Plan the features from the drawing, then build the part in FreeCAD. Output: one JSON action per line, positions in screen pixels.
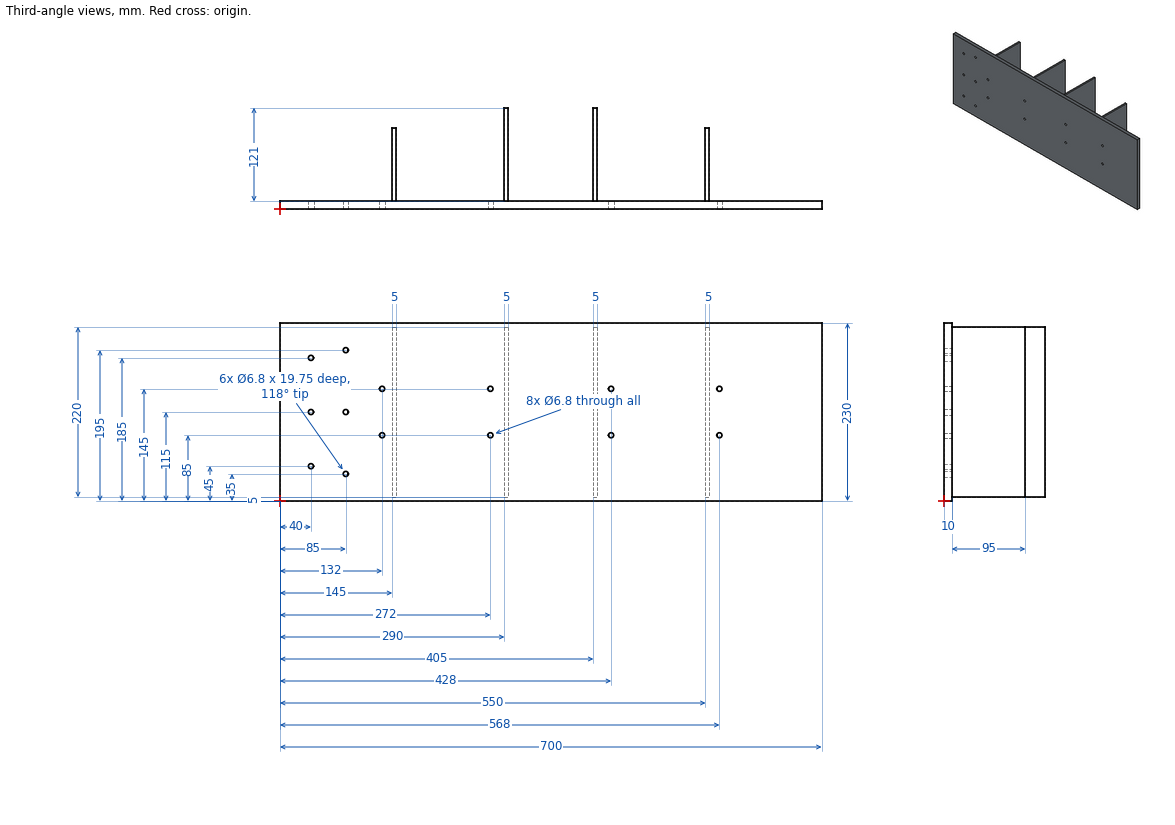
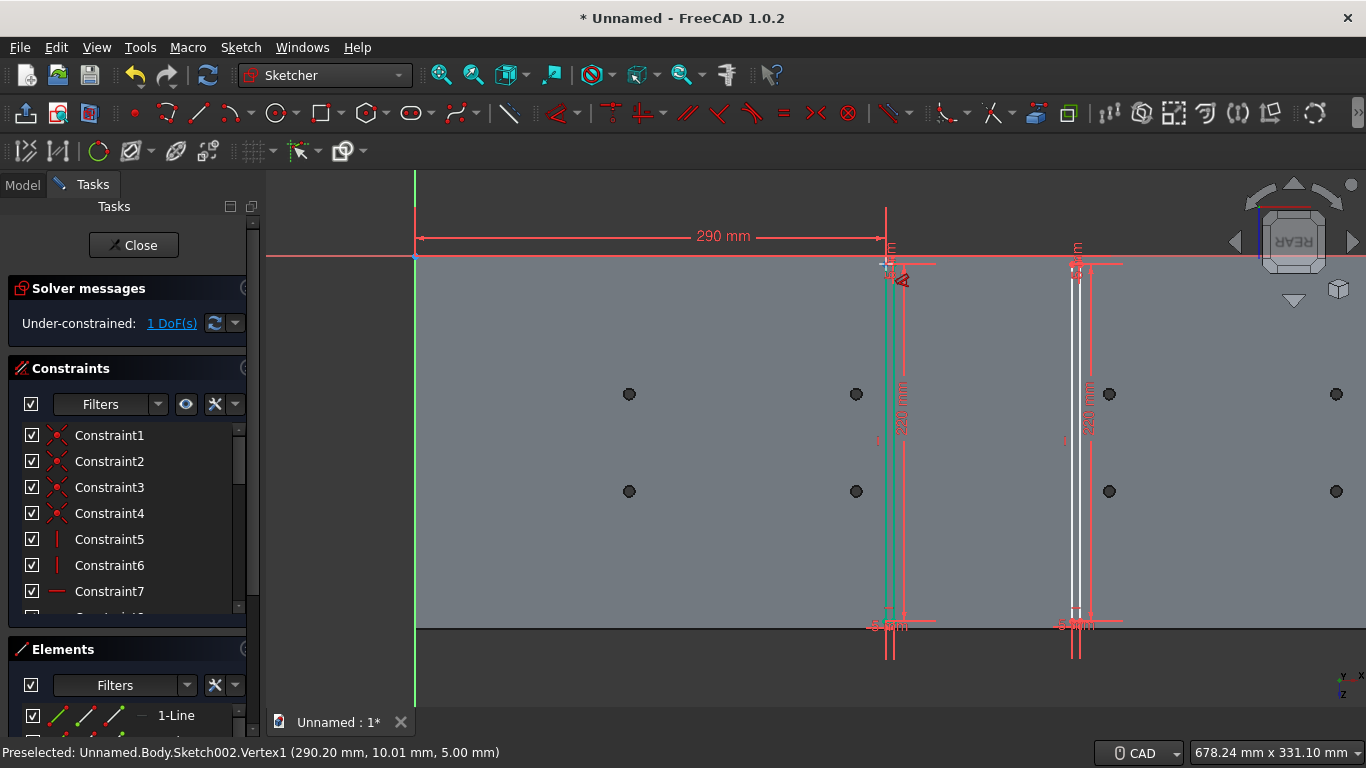
{"action": "scroll", "coordinate": [1072, 264], "scroll_direction": "up", "scroll_amount": 3}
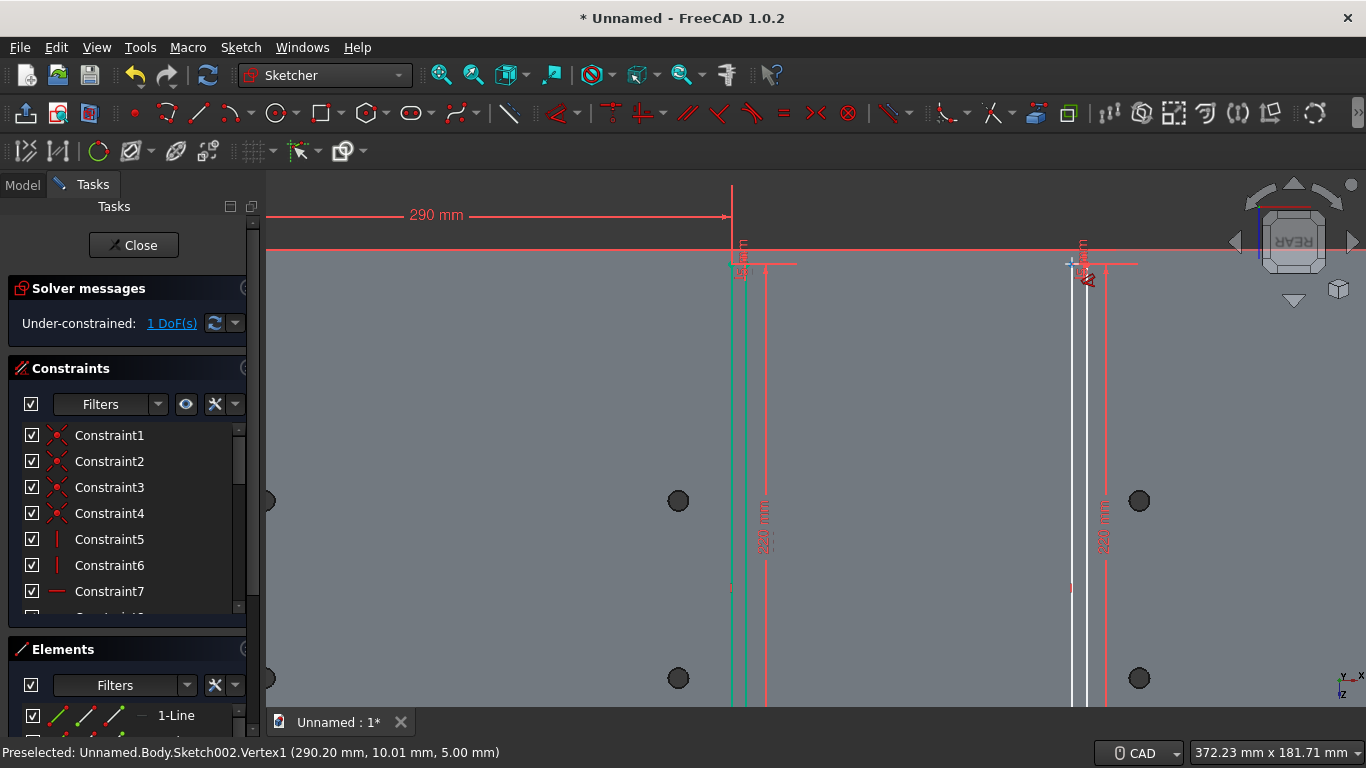
{"action": "left_click", "coordinate": [1072, 264]}
{"action": "left_click", "coordinate": [683, 216]}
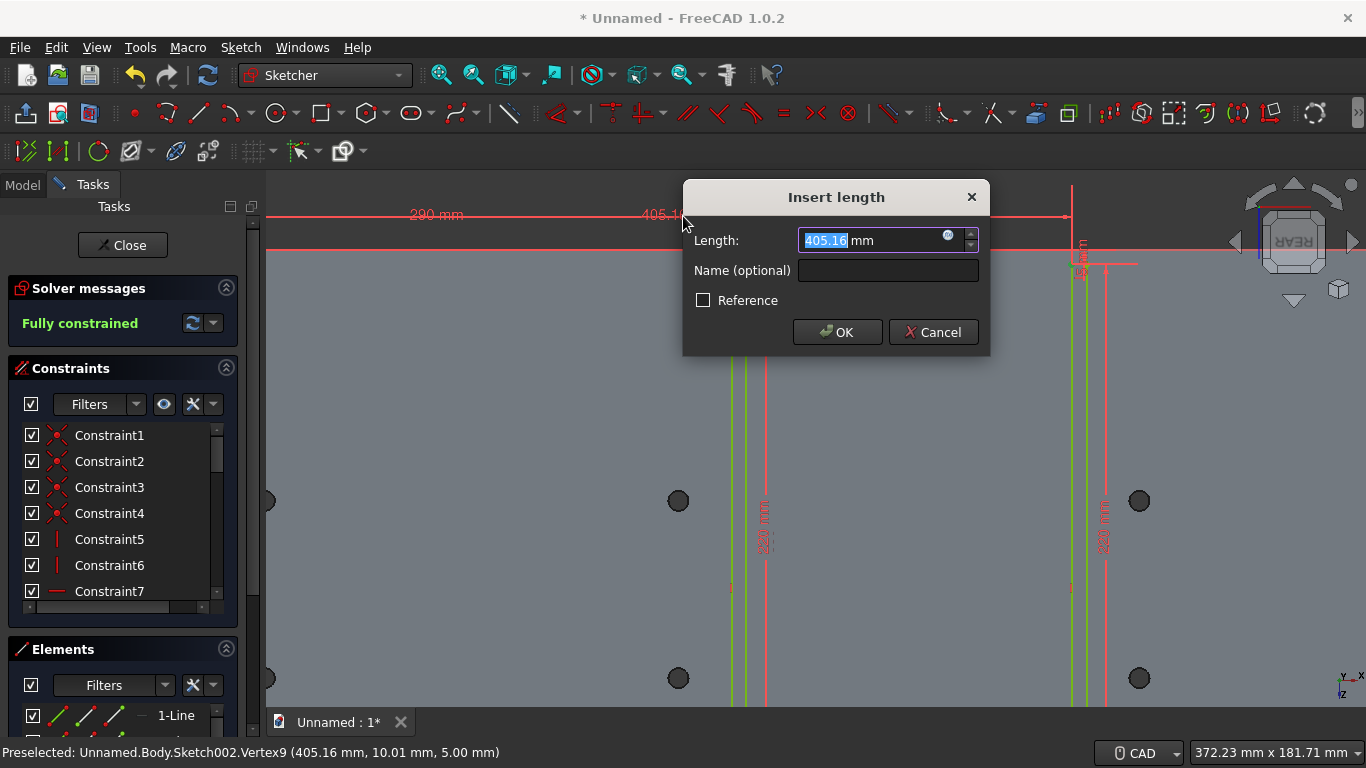
{"action": "type", "text": "405"}
{"action": "key", "text": "Return"}
{"action": "key", "text": "Escape"}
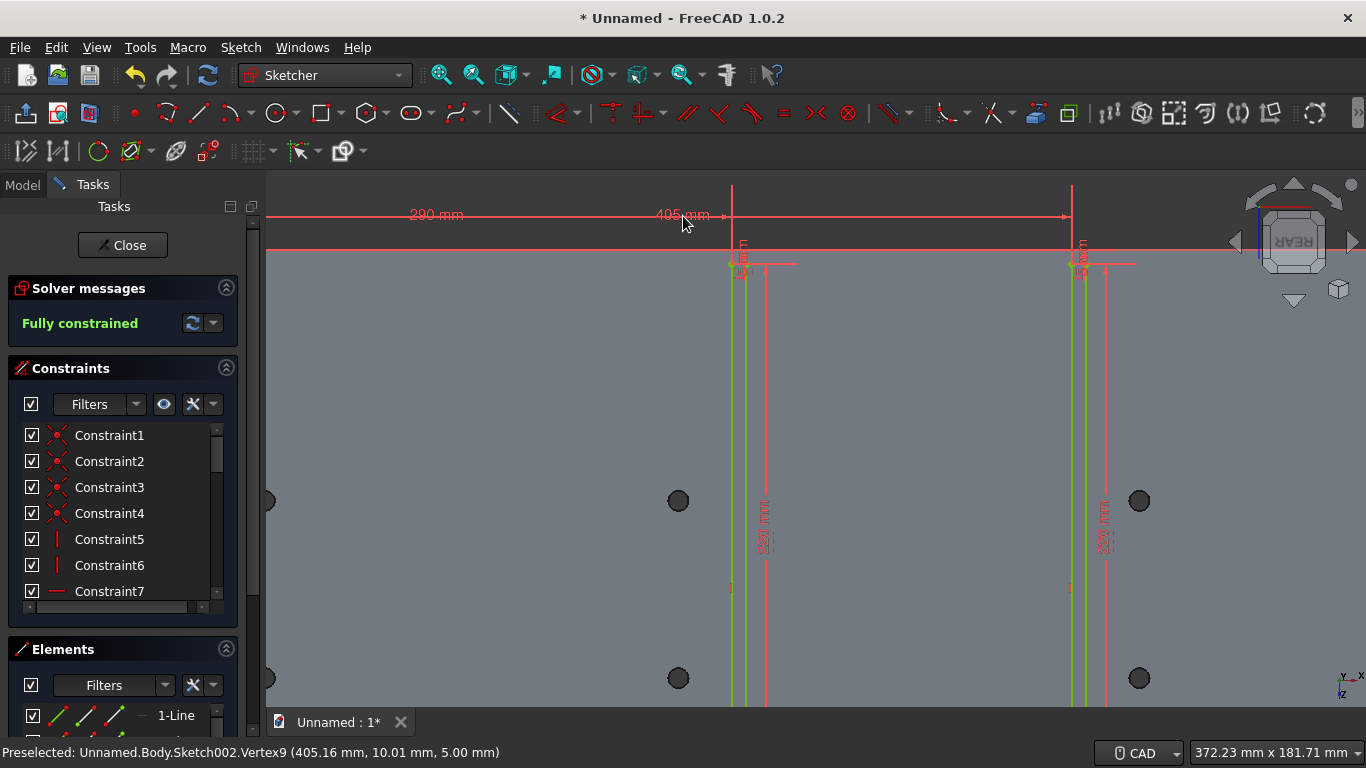
{"action": "left_click", "coordinate": [123, 245]}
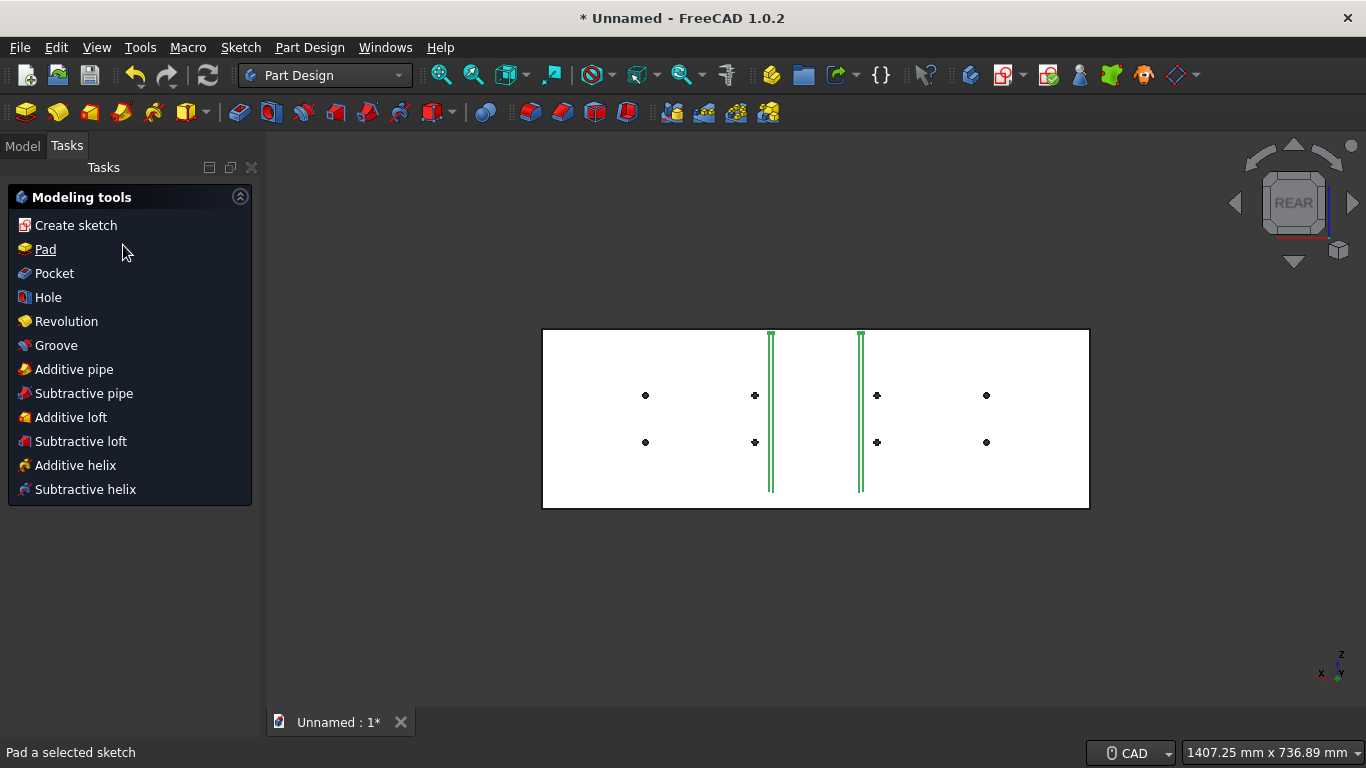
{"action": "left_click", "coordinate": [26, 112]}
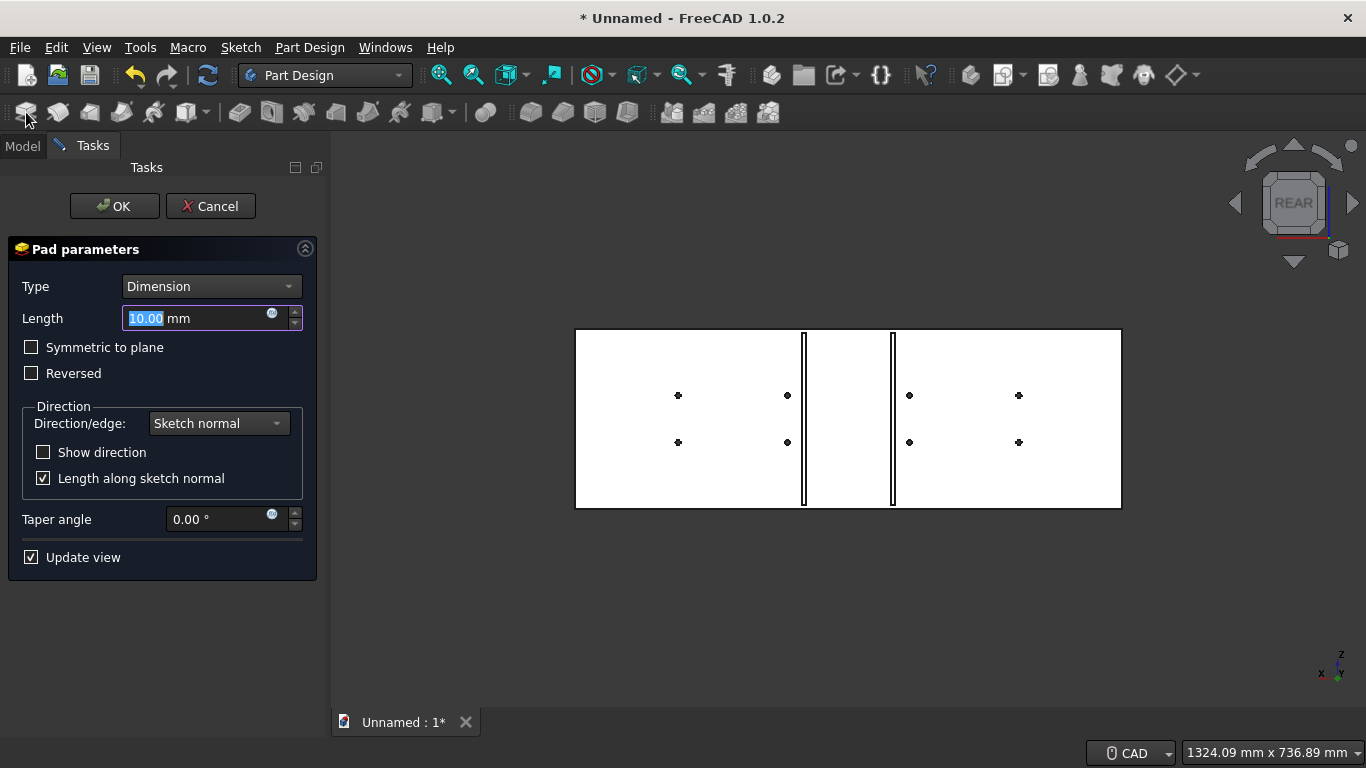
{"action": "type", "text": "121"}
{"action": "key", "text": "Tab"}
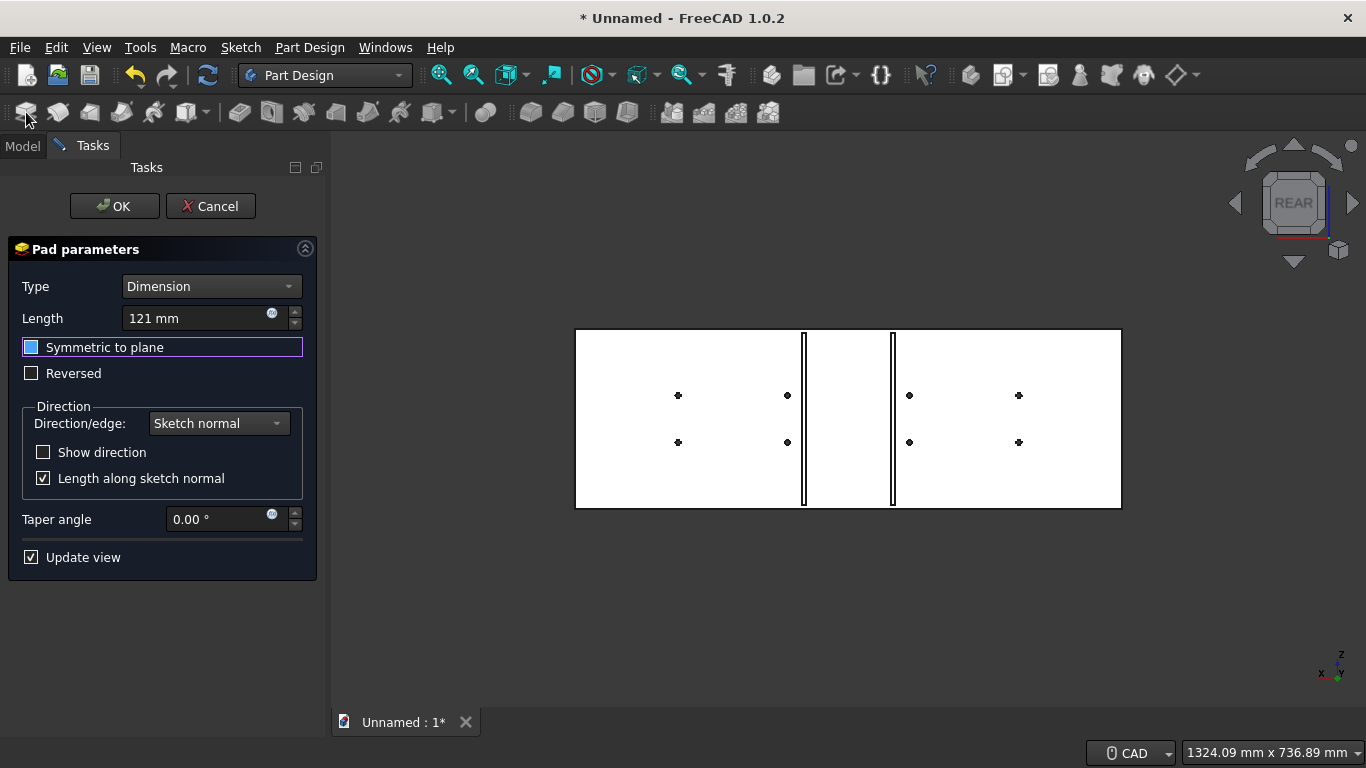
{"action": "left_click", "coordinate": [115, 206]}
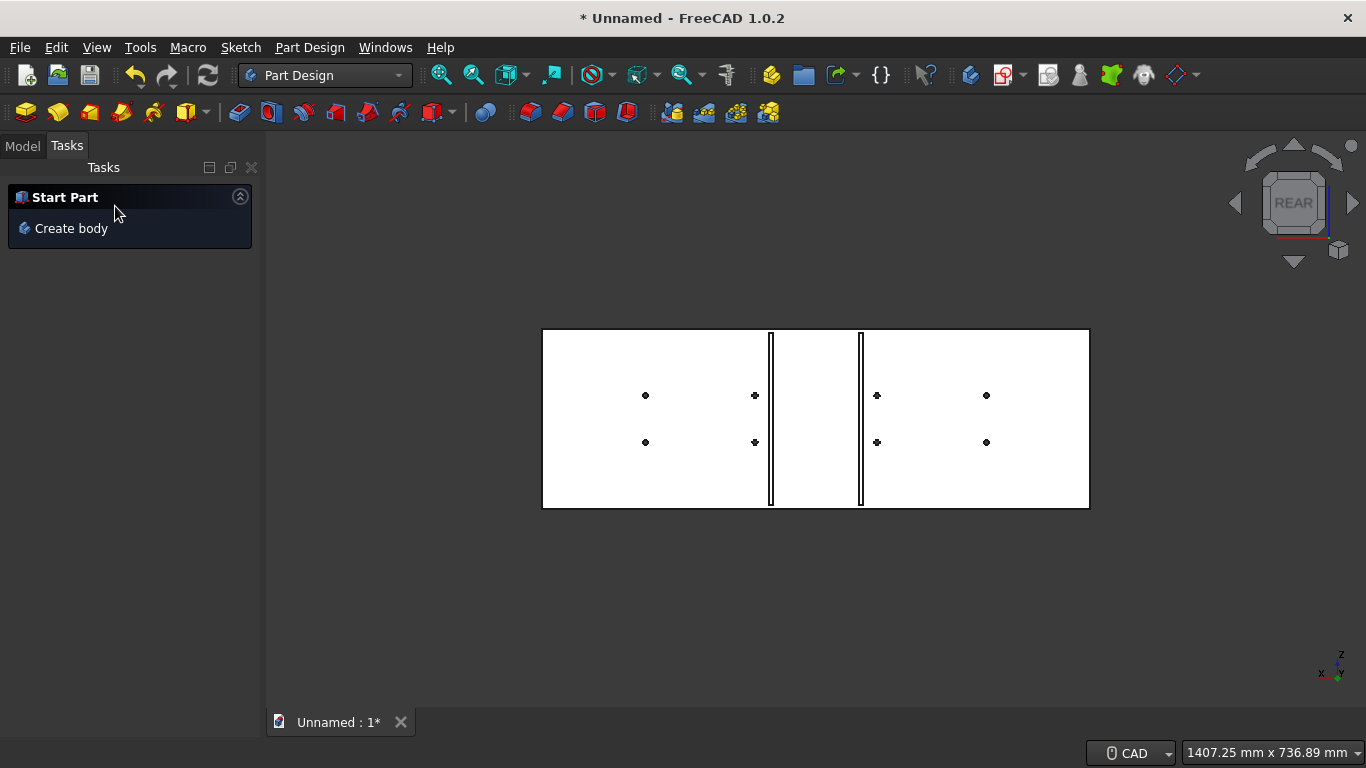
{"action": "left_click", "coordinate": [816, 392]}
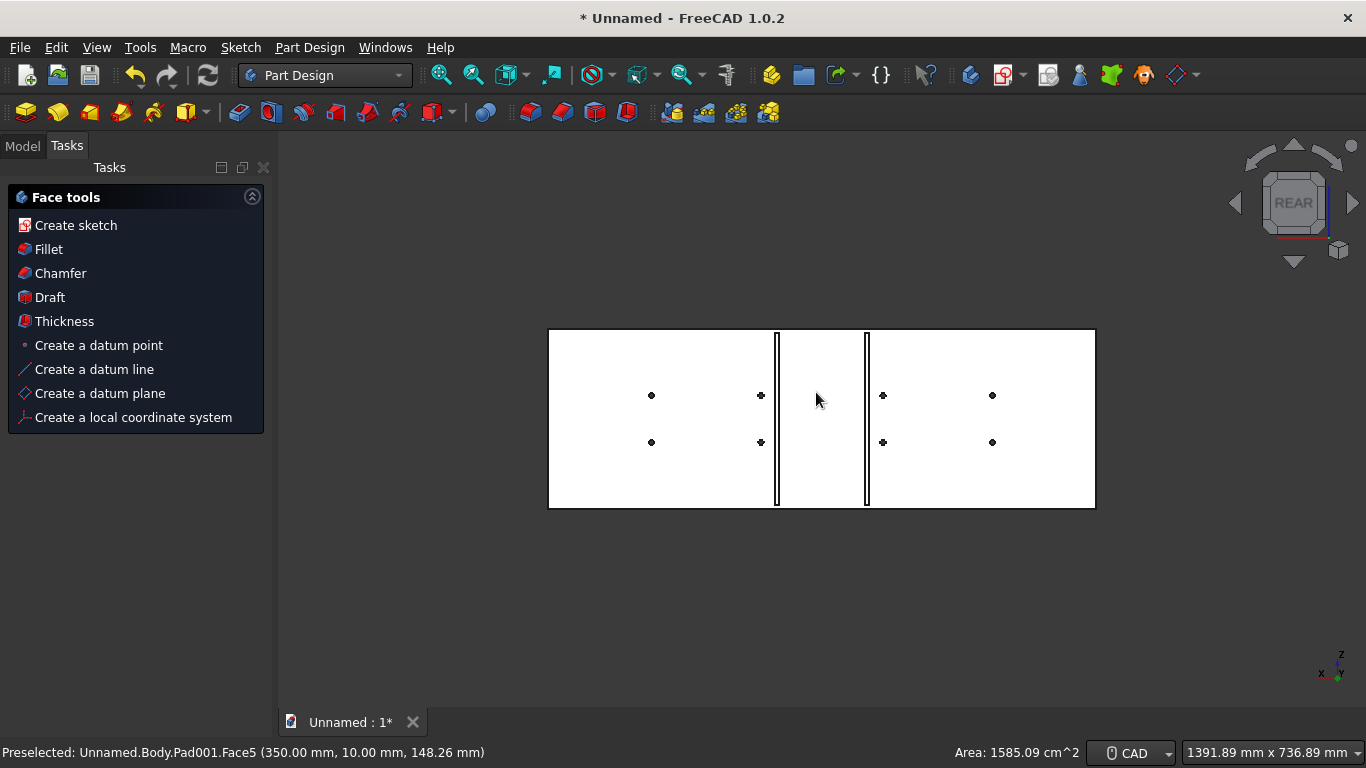
{"action": "left_click", "coordinate": [1004, 76]}